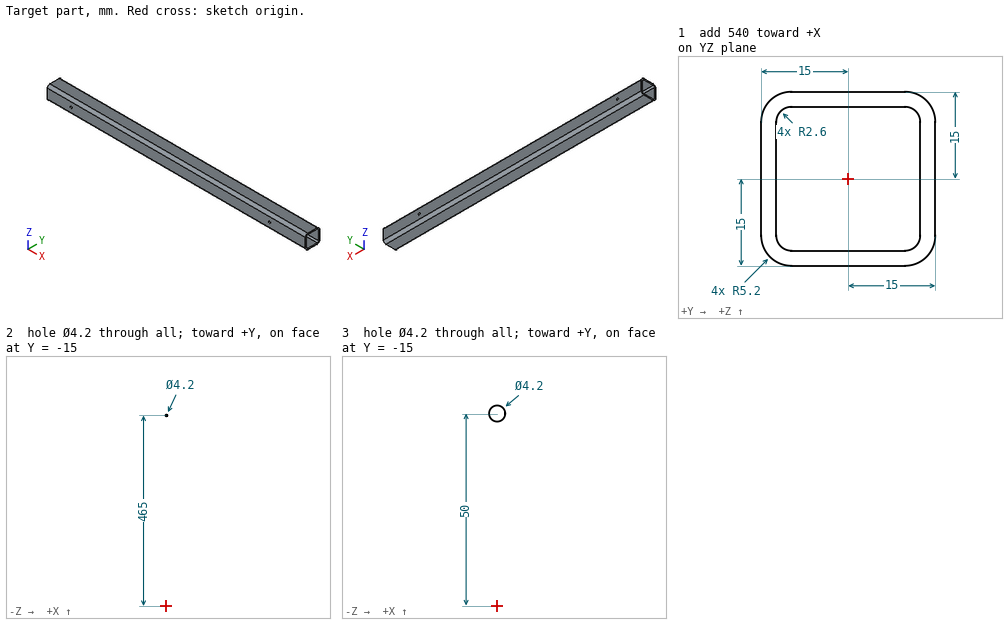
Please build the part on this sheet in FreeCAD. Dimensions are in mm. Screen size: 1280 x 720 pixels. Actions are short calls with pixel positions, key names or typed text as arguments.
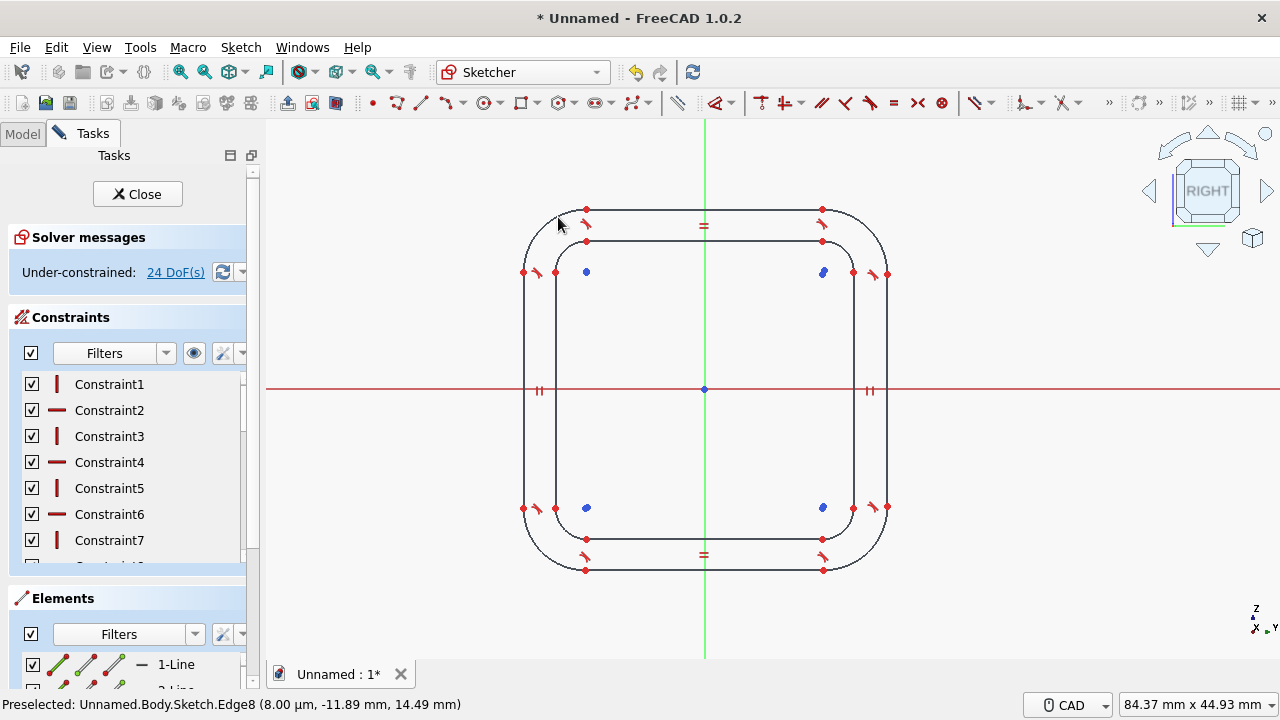
click(556, 438)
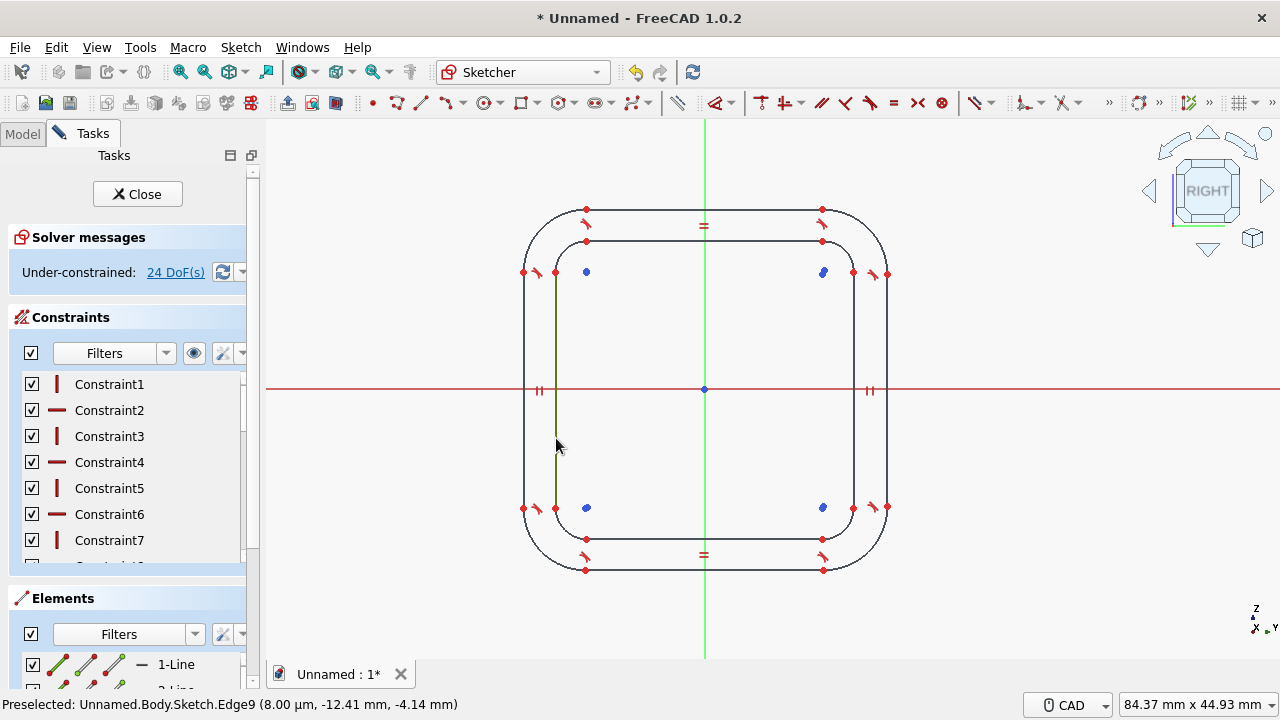
click(573, 245)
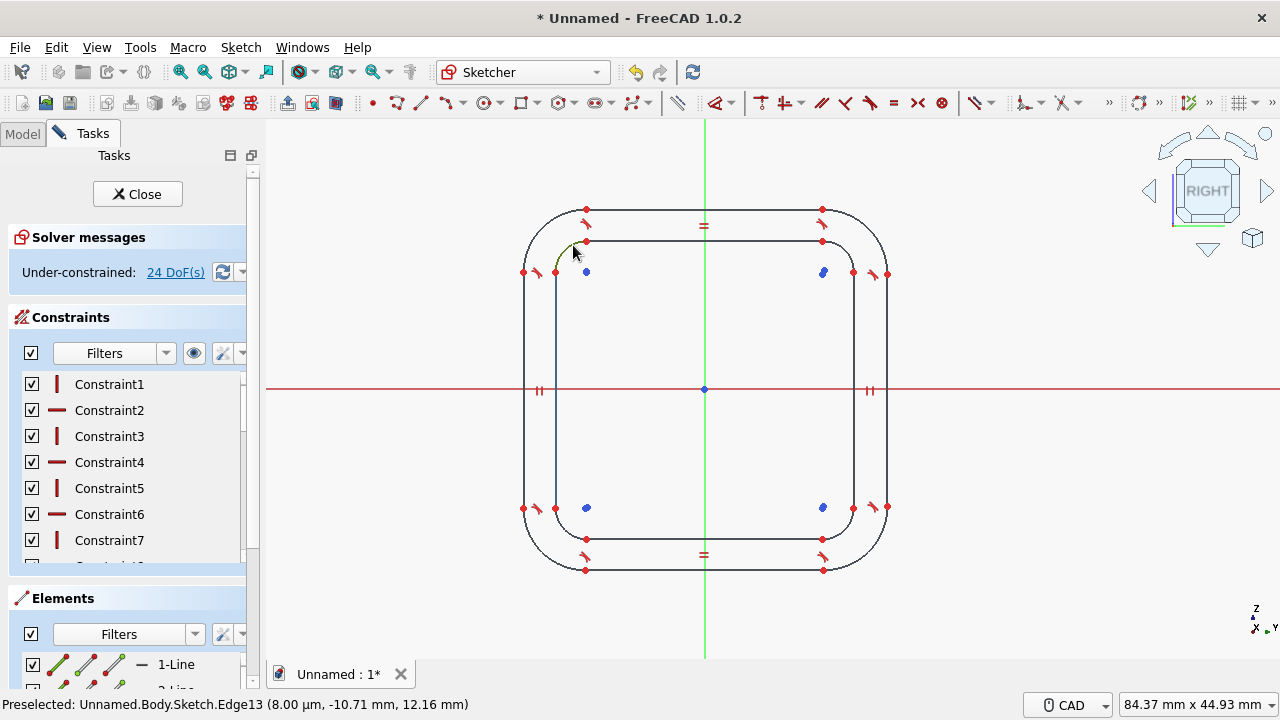
click(870, 104)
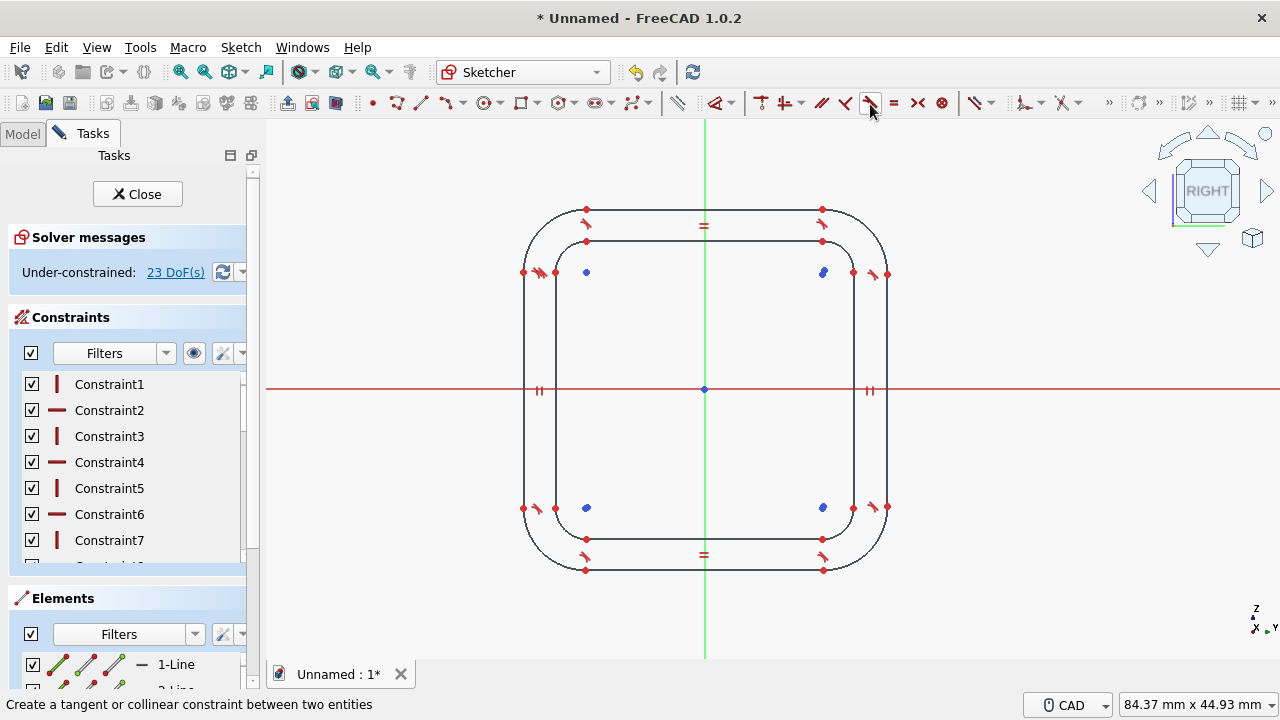
click(556, 438)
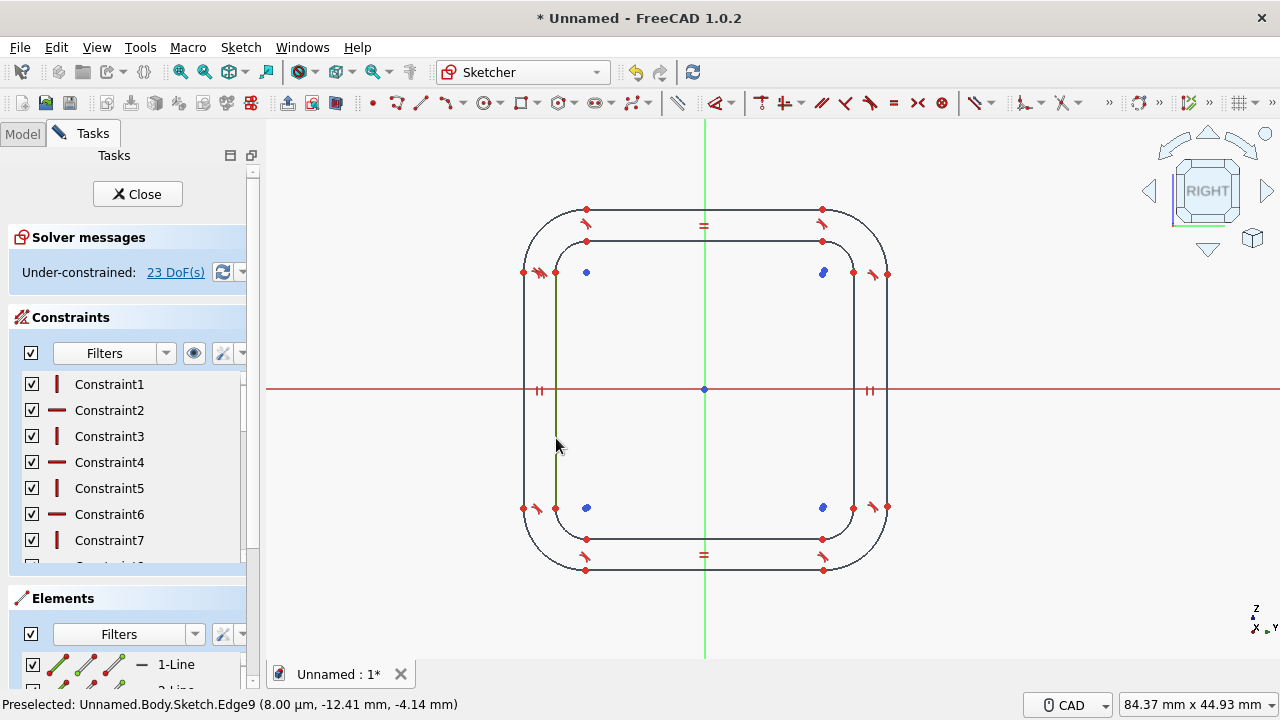
click(559, 522)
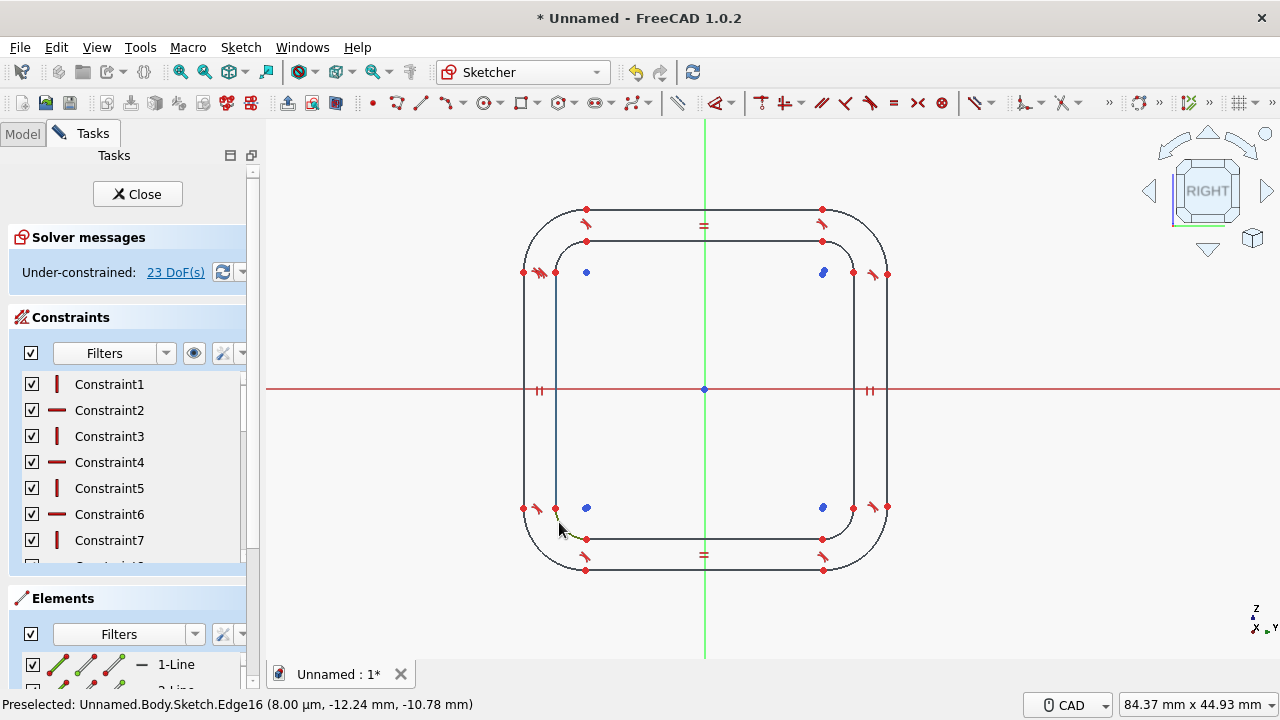
click(870, 104)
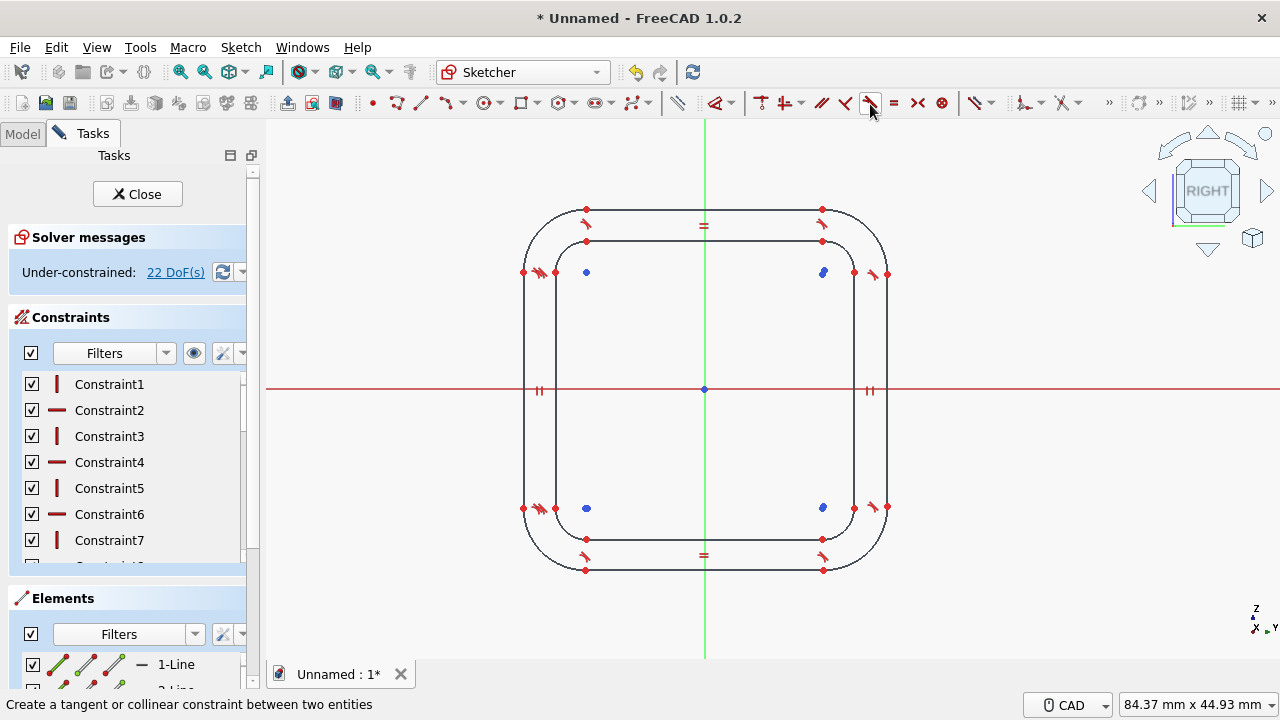
click(657, 241)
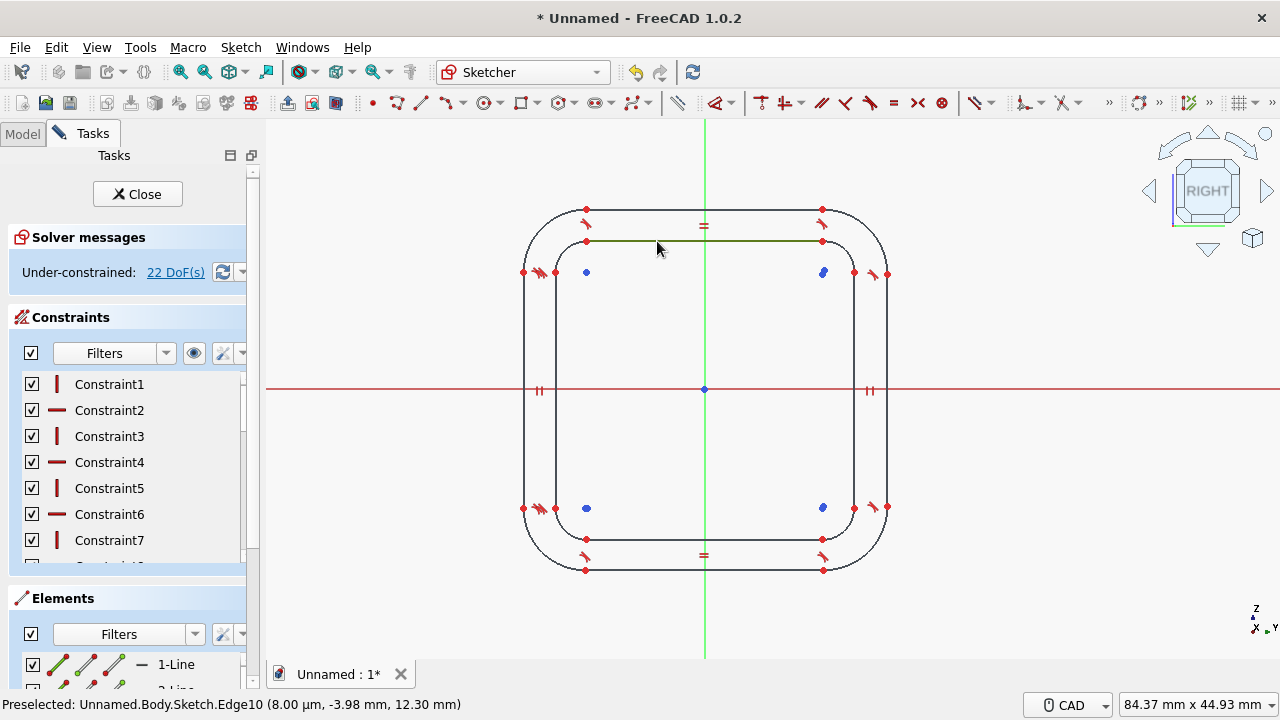
click(573, 245)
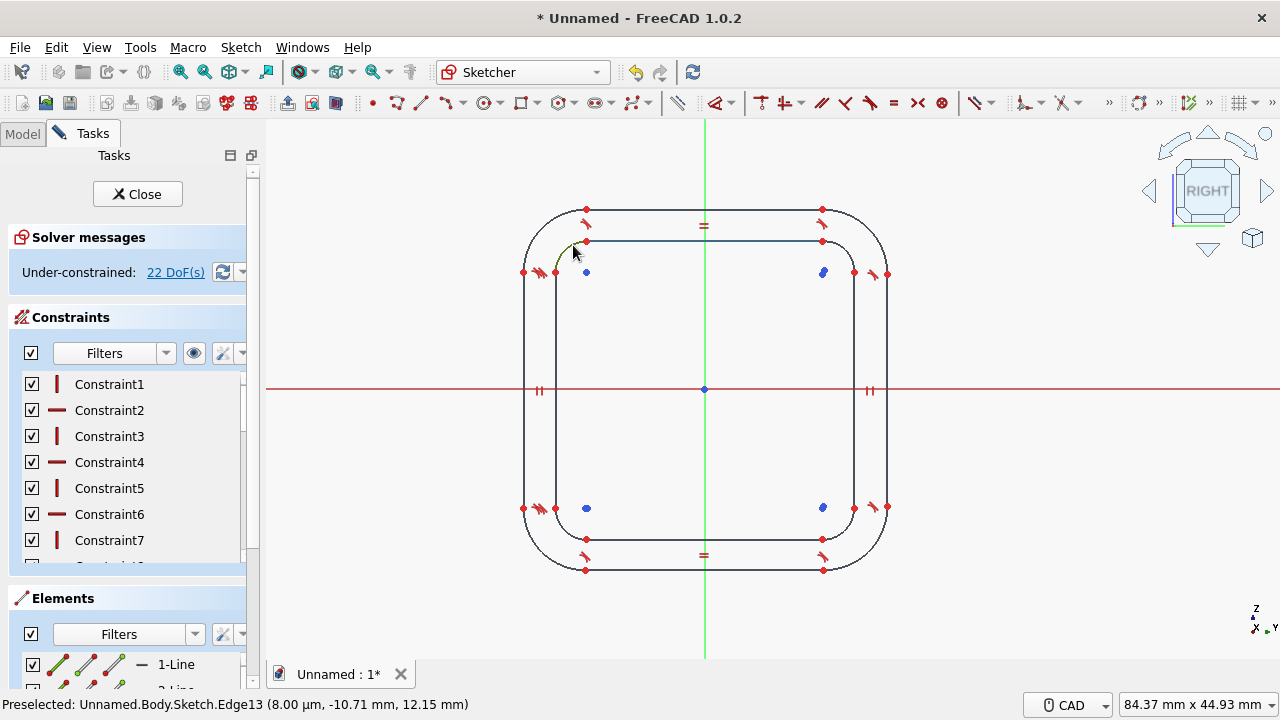
click(870, 104)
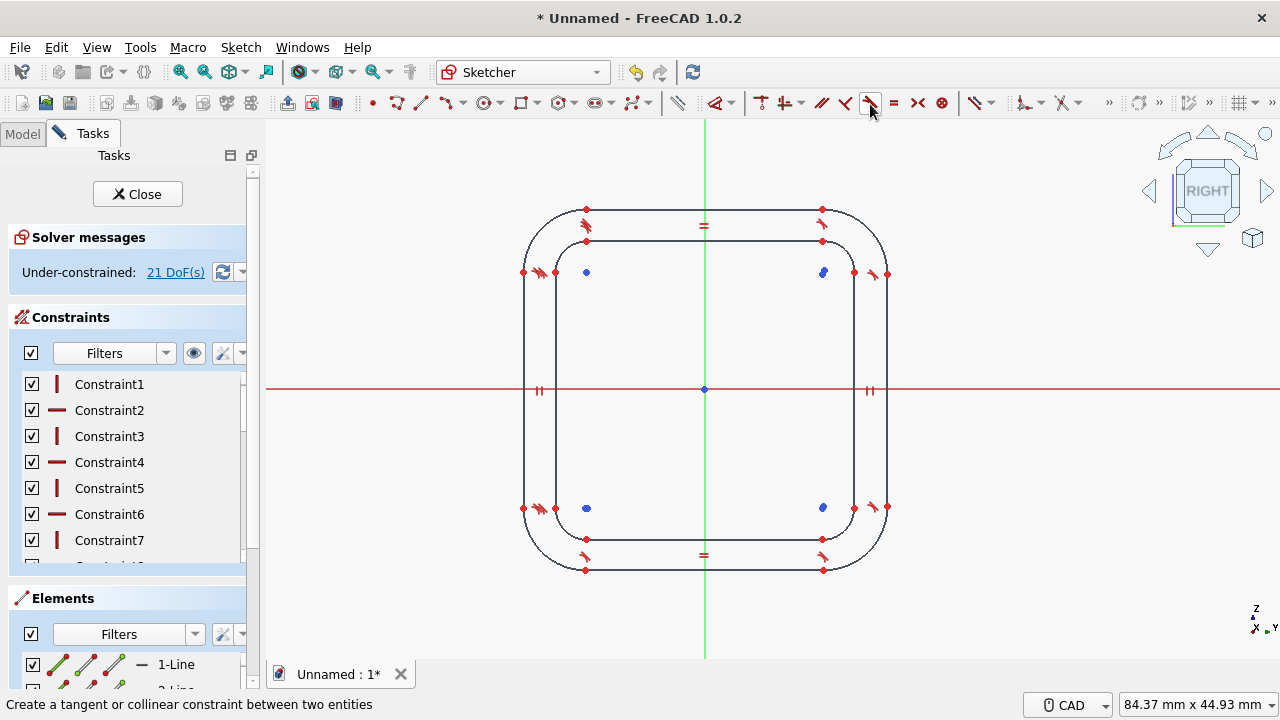
click(657, 241)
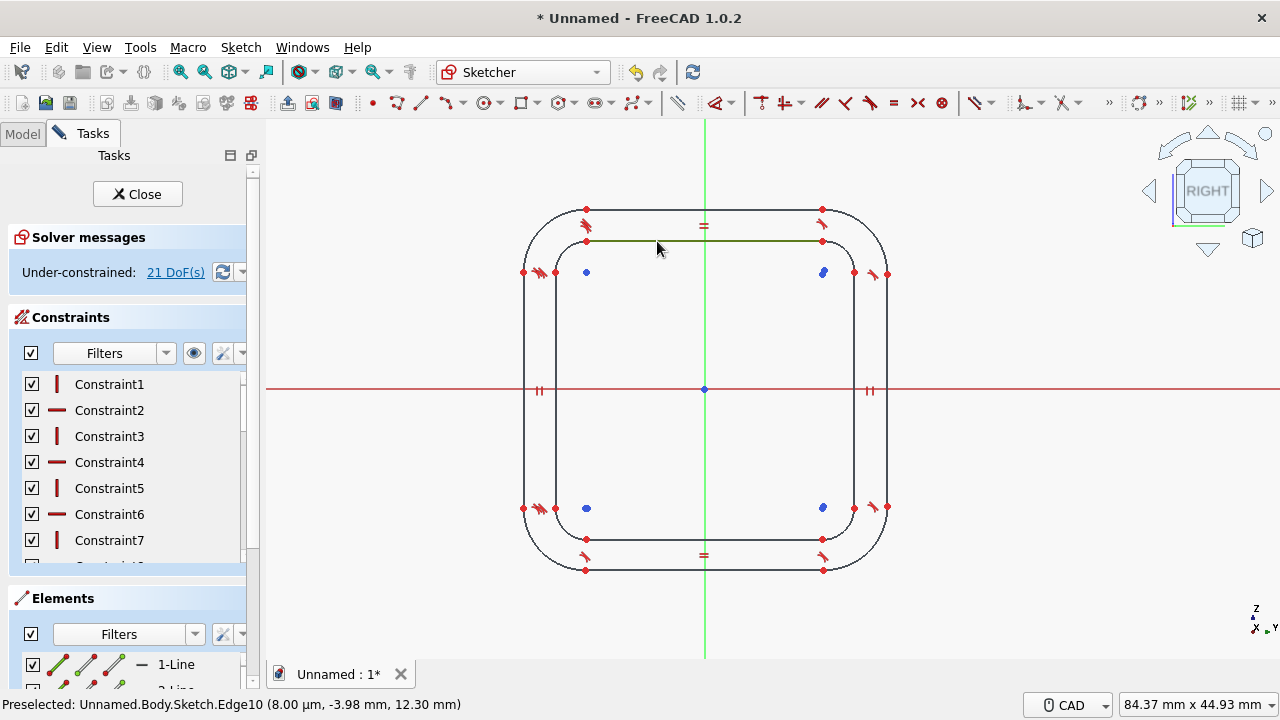
click(851, 258)